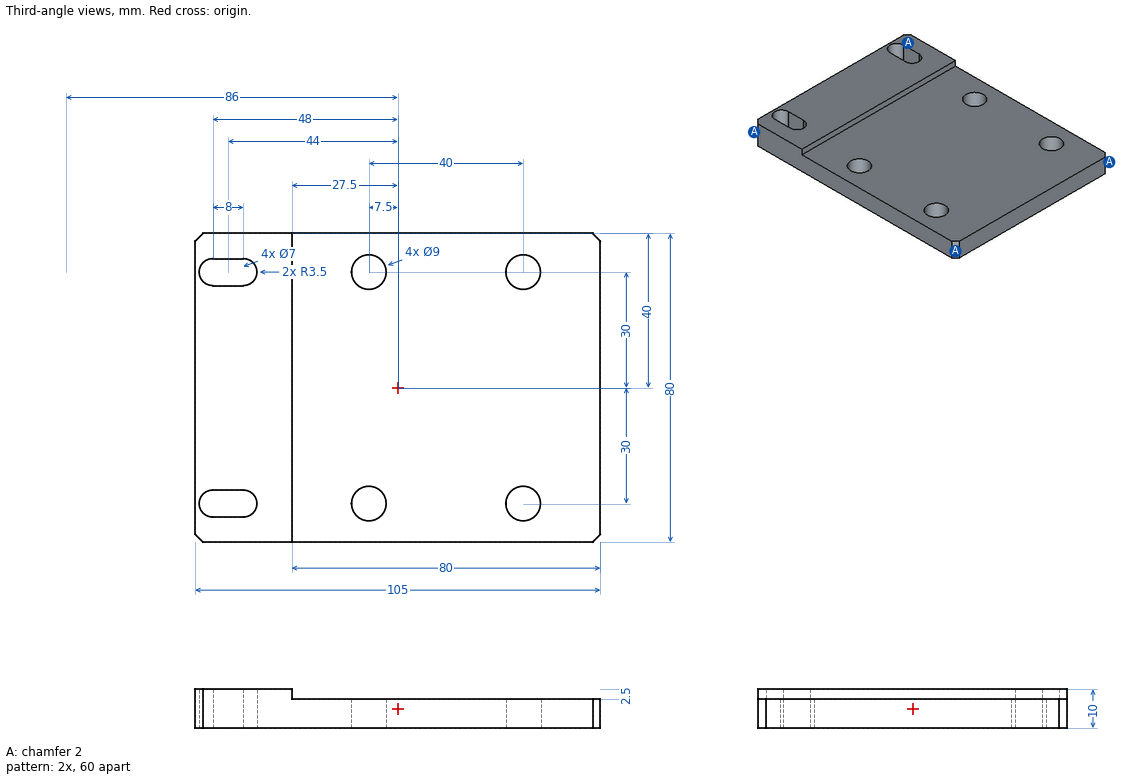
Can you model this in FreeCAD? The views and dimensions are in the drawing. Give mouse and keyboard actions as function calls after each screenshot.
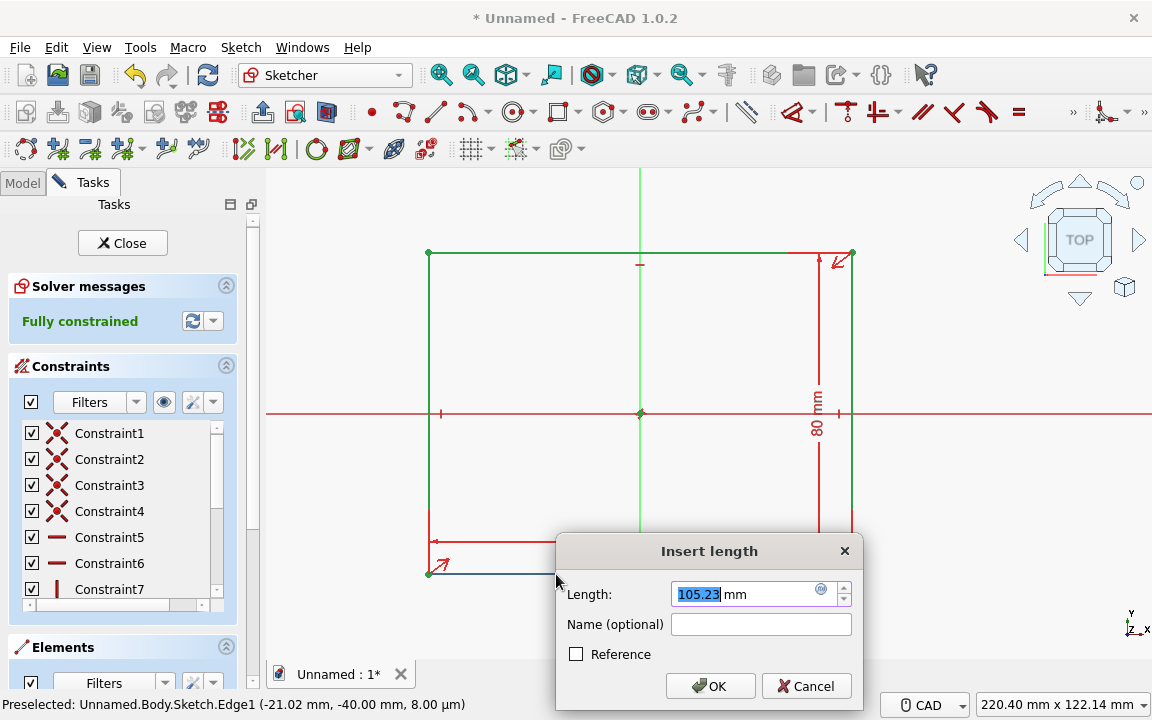
text(105)
key(Return)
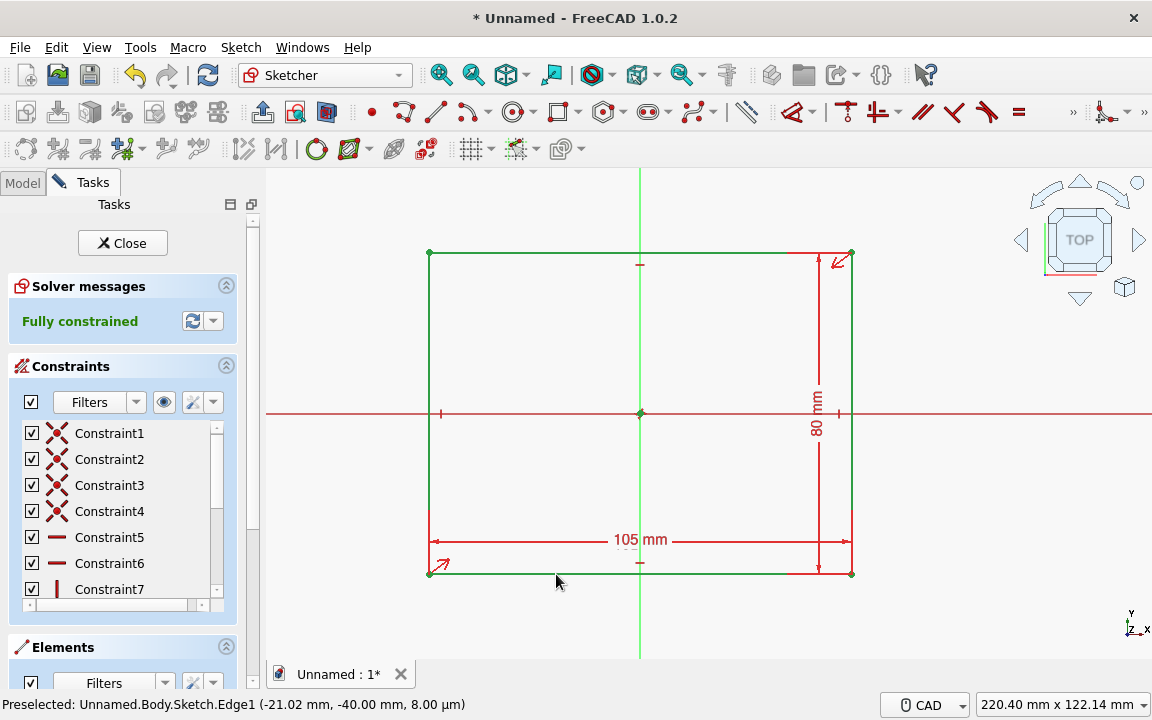
click(123, 243)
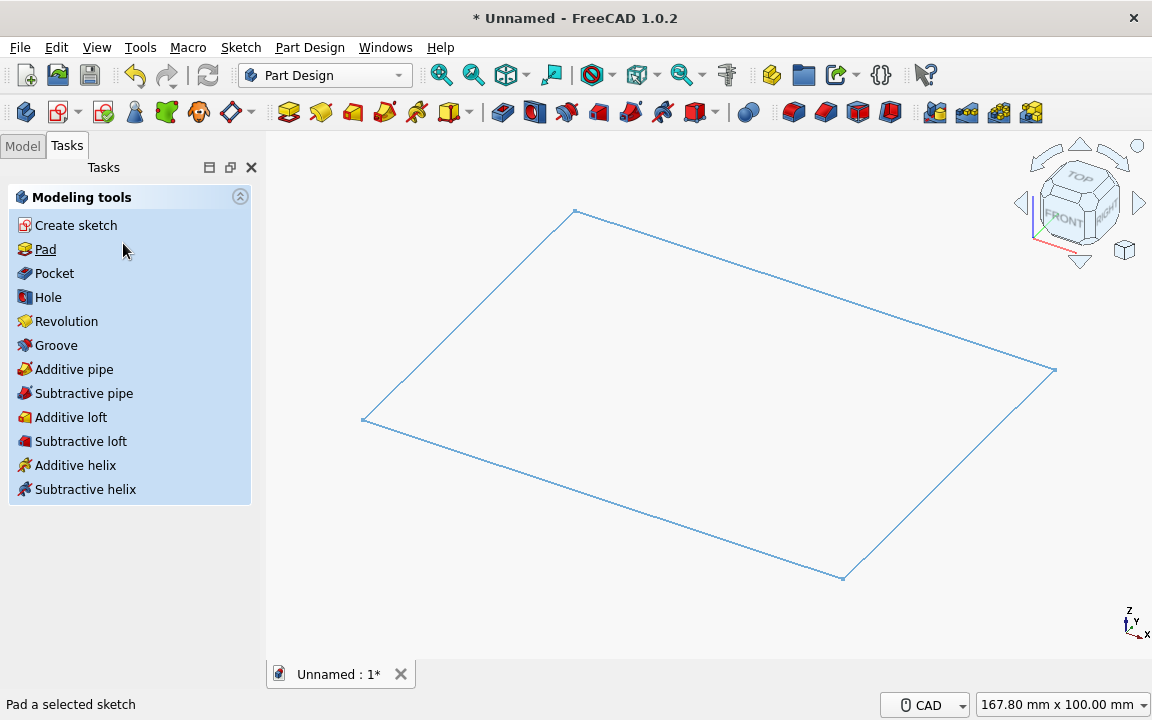
click(290, 112)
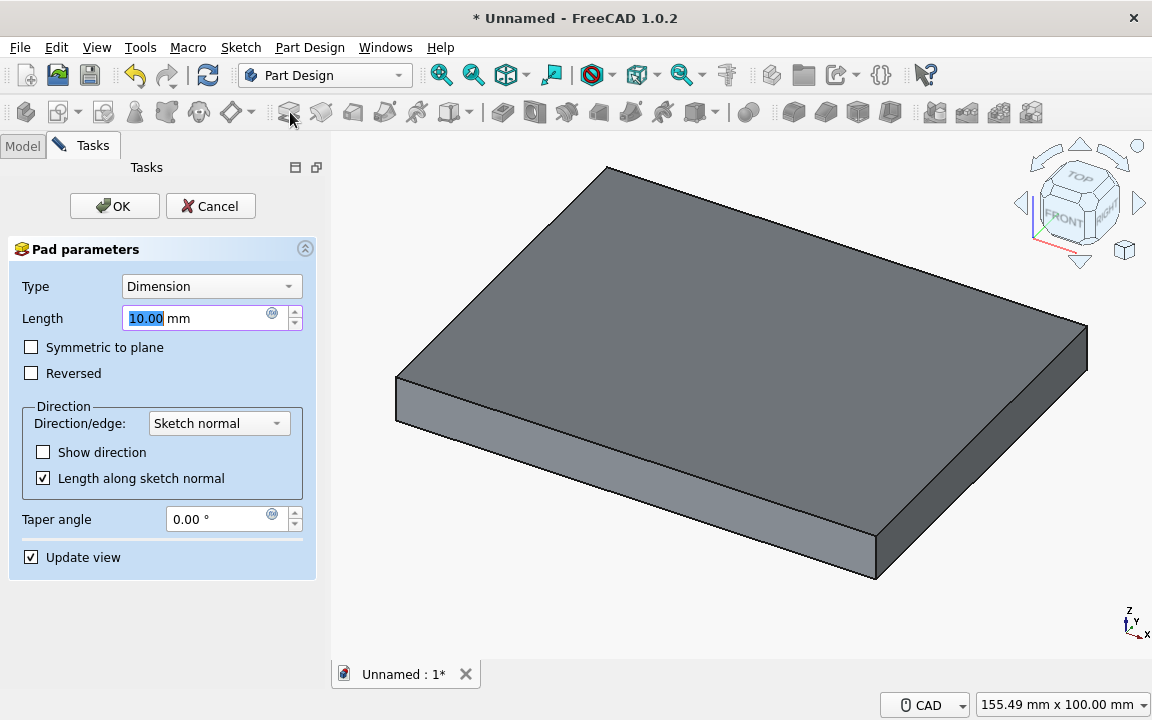
text(10)
key(Tab)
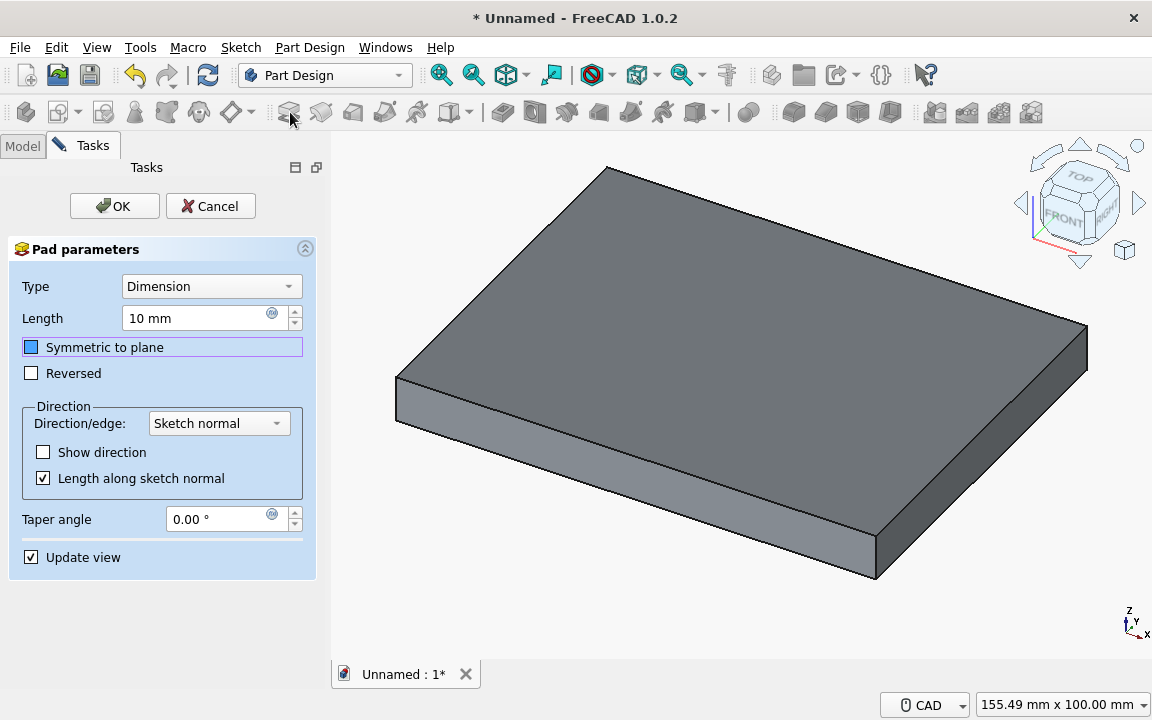
click(30, 347)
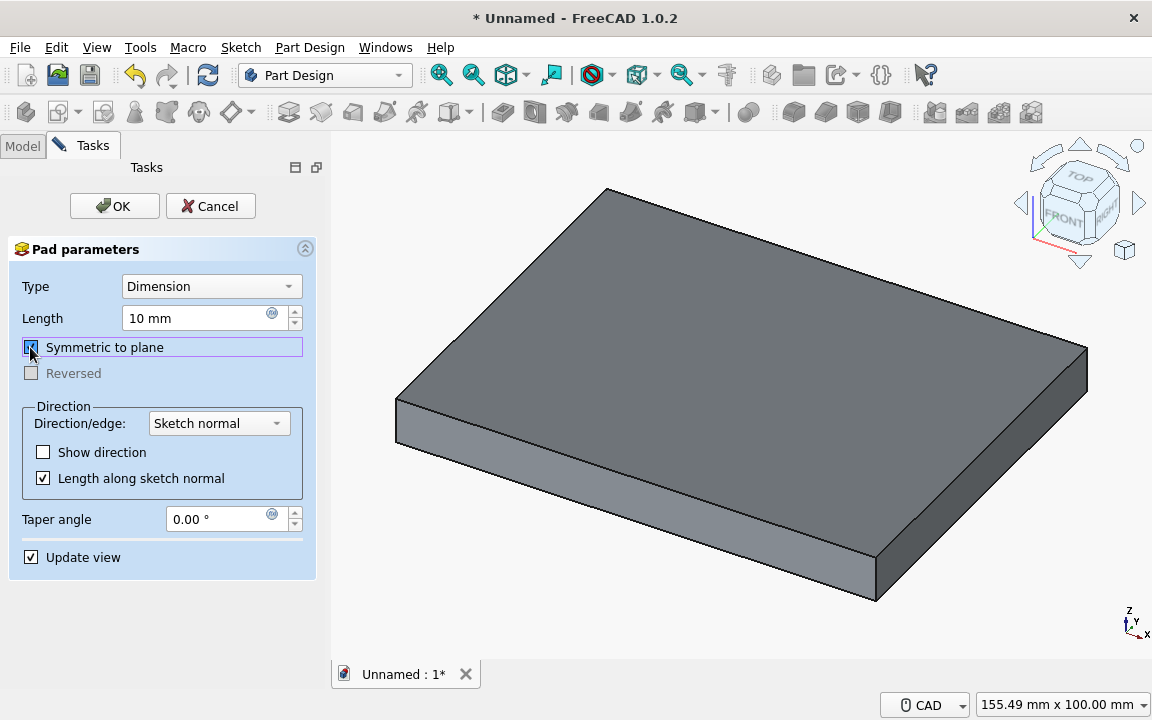
click(115, 206)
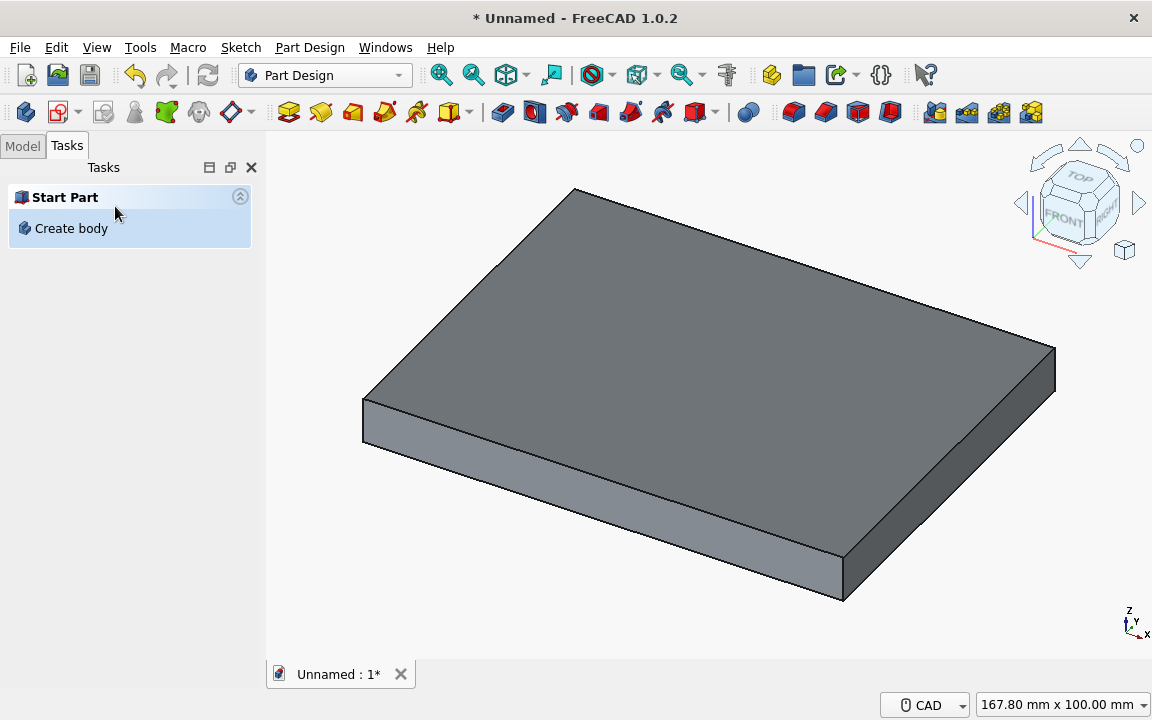
click(709, 372)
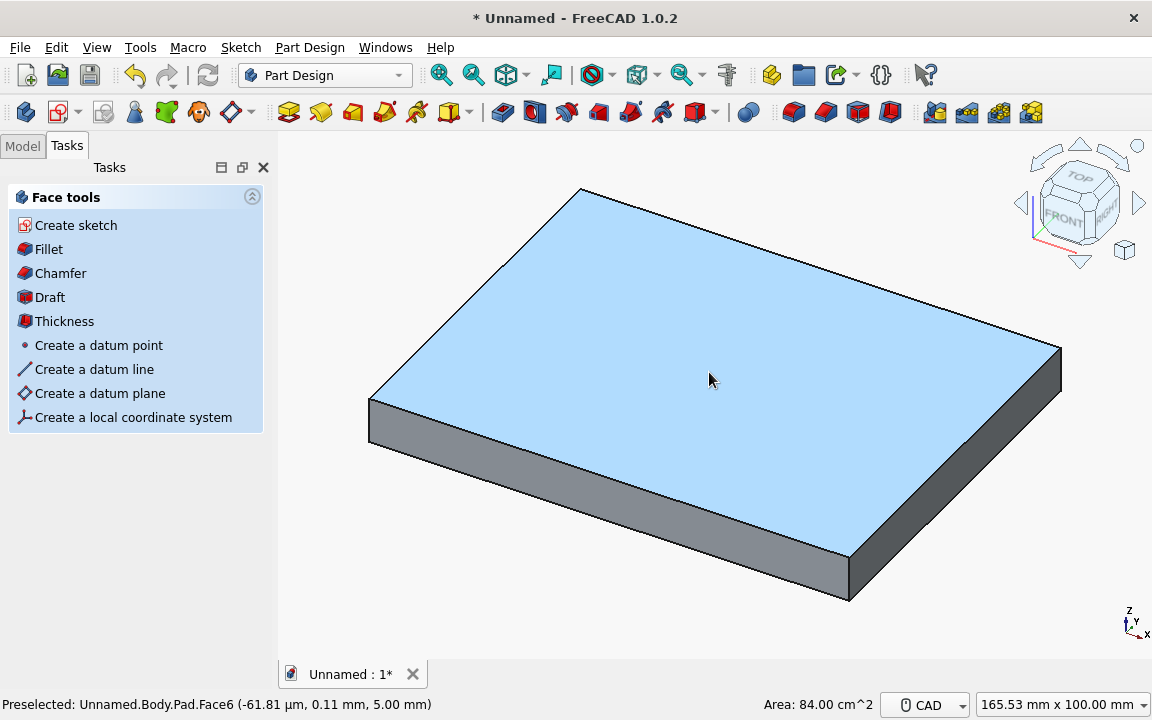
click(58, 112)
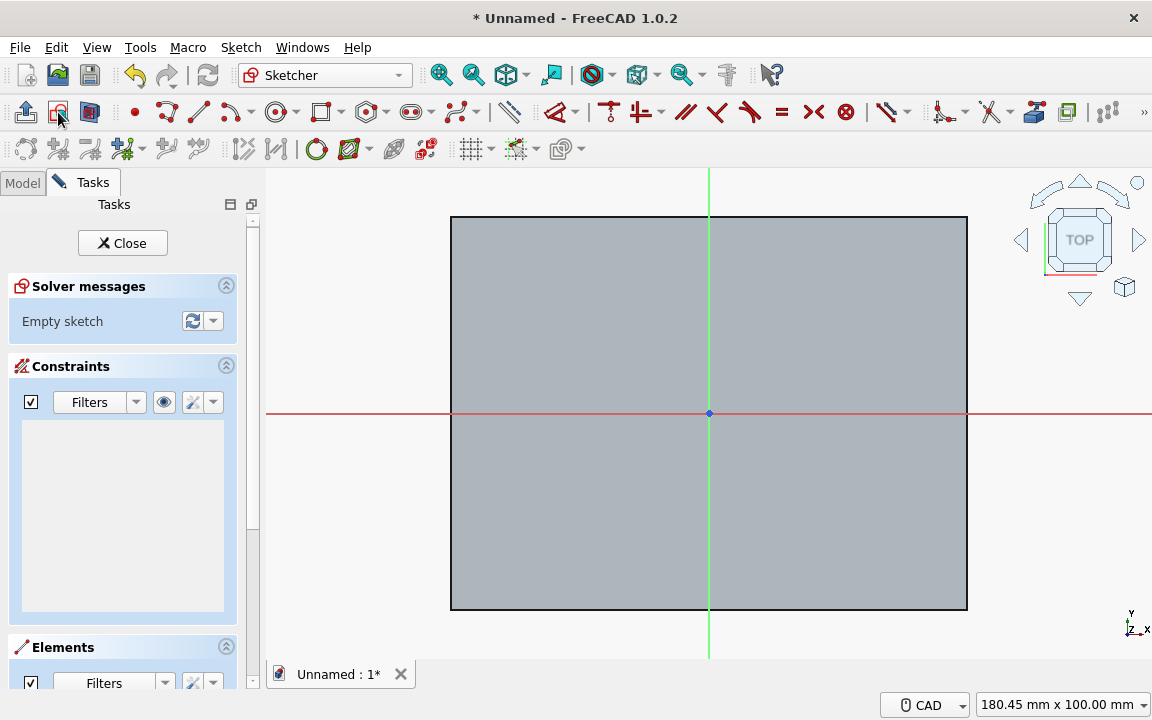
scroll(294, 413, down, 1)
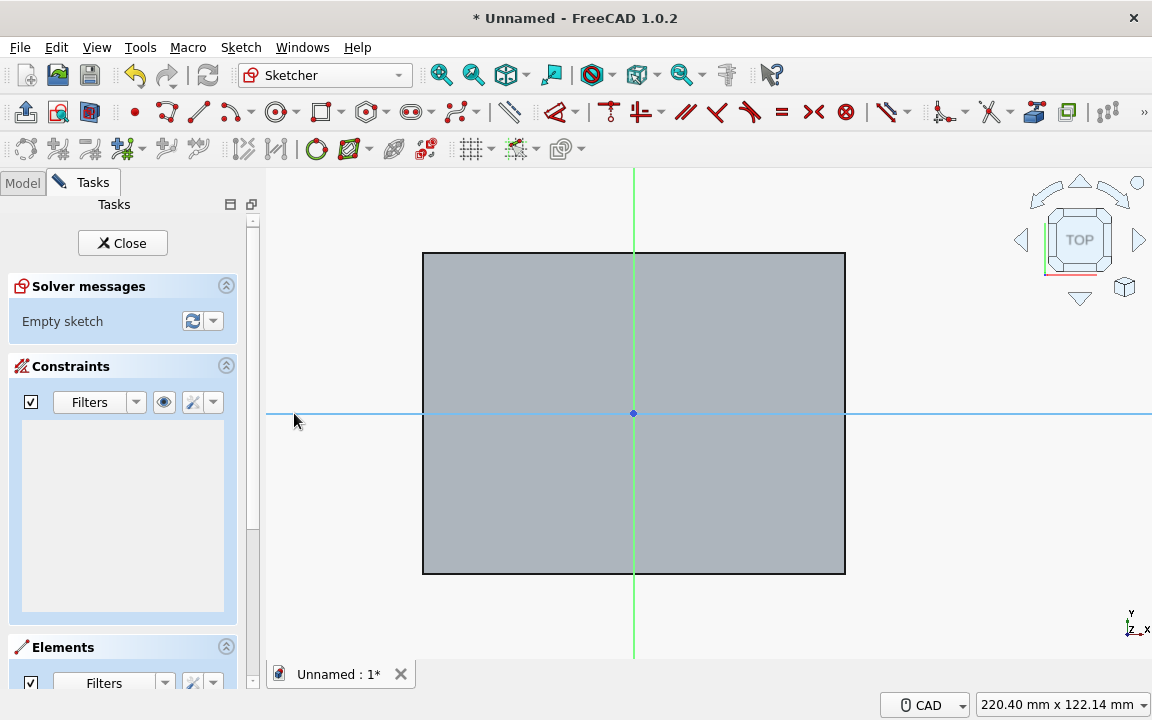
click(322, 112)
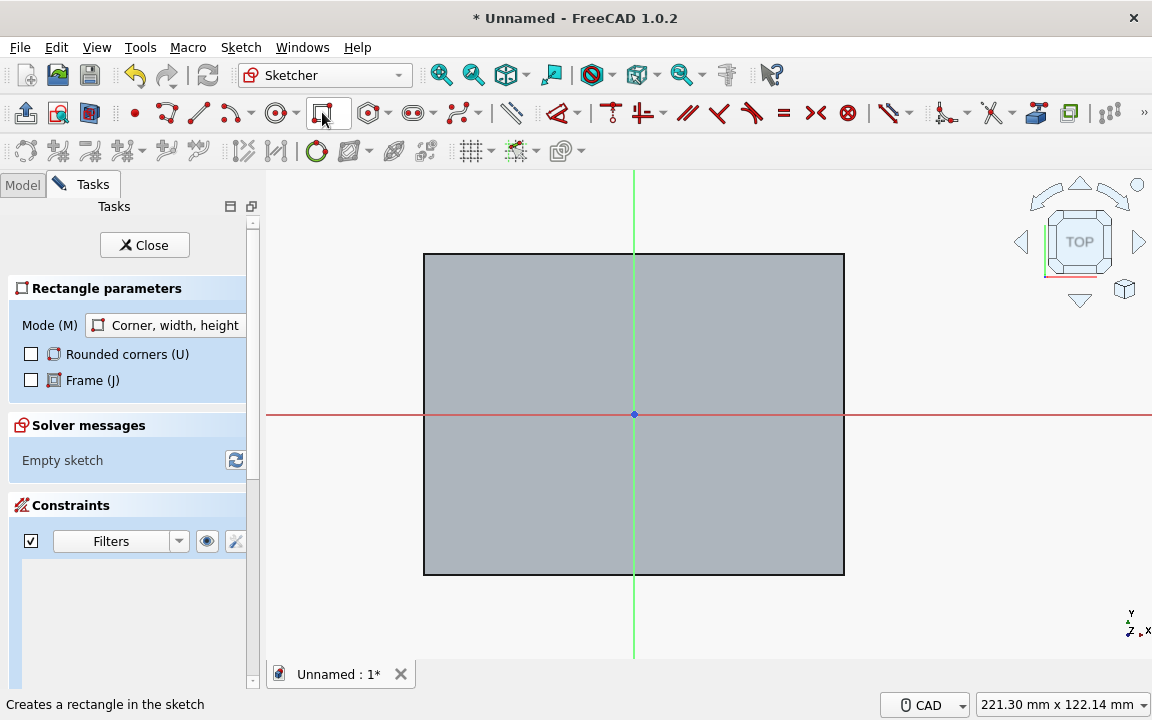
click(524, 254)
click(844, 575)
key(Escape)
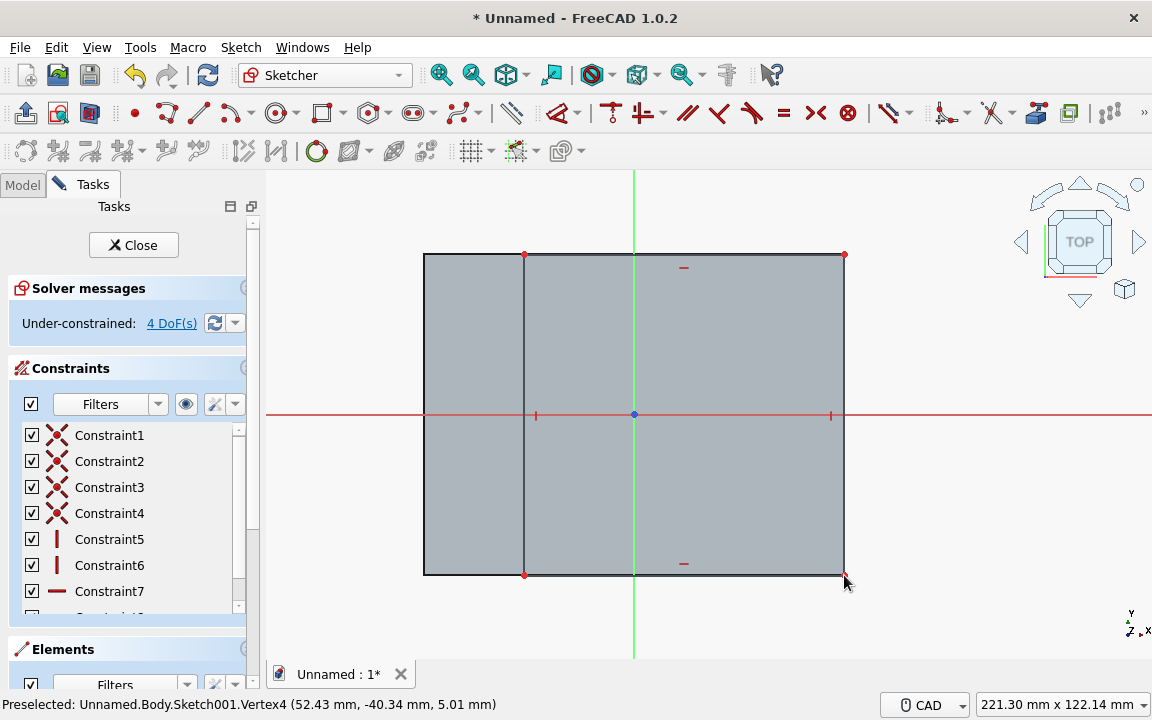
click(524, 351)